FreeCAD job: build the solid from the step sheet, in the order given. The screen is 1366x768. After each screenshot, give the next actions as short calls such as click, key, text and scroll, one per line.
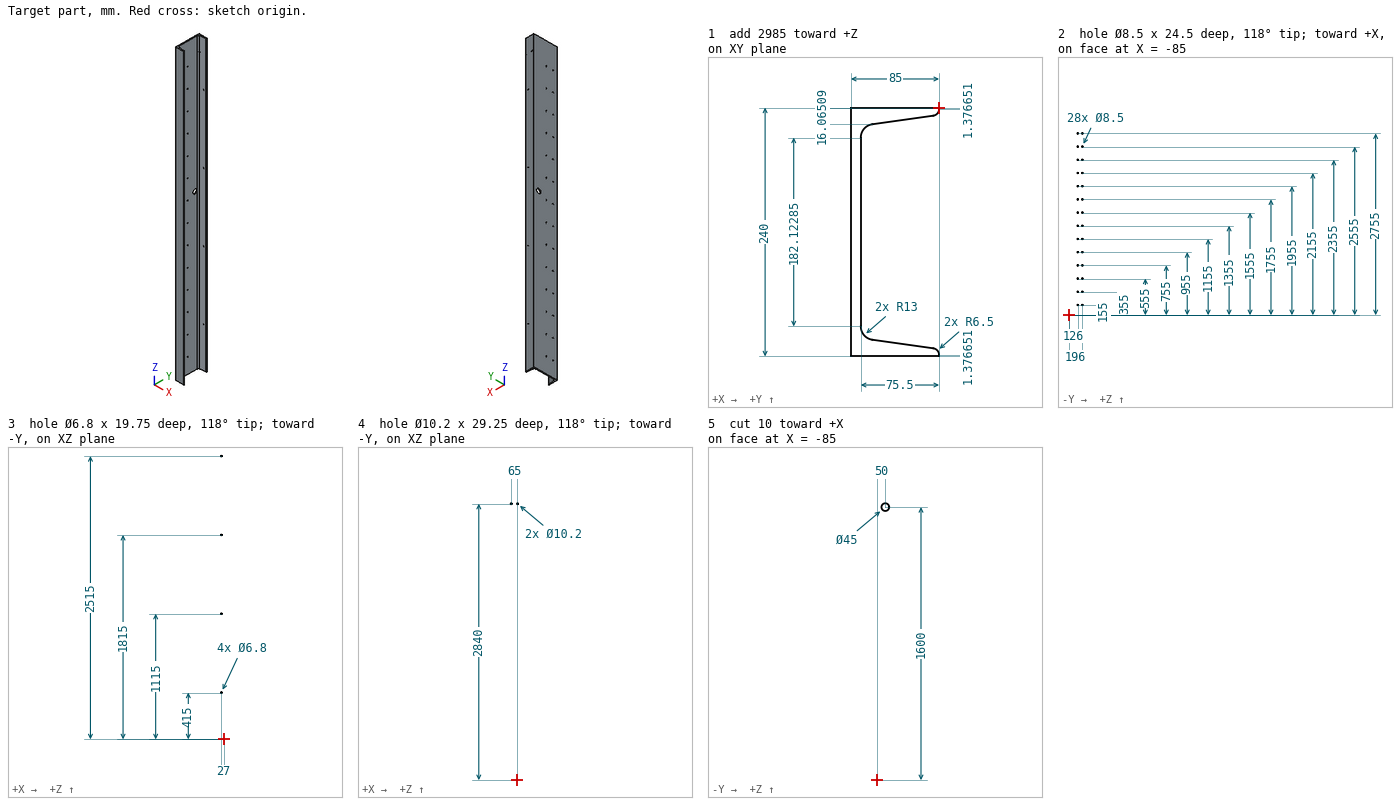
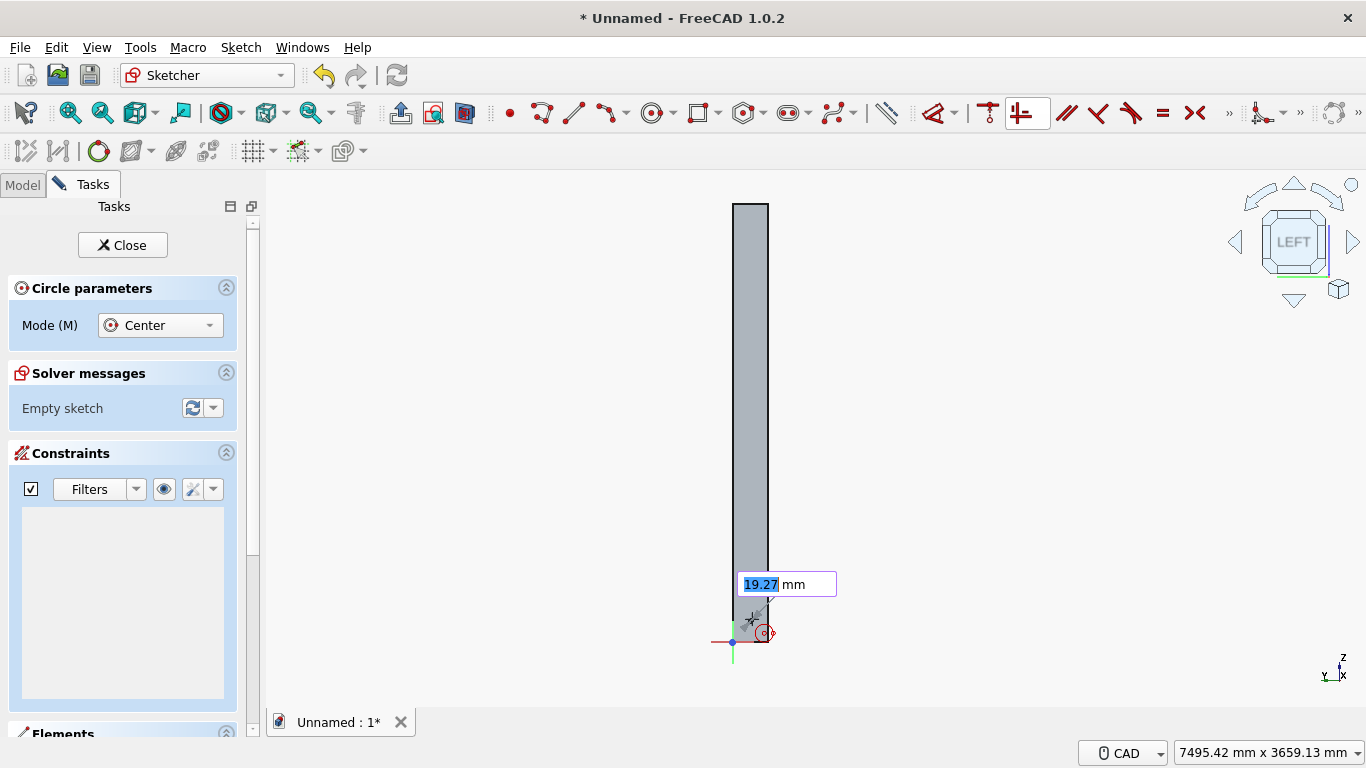
text(8.5)
key(Return)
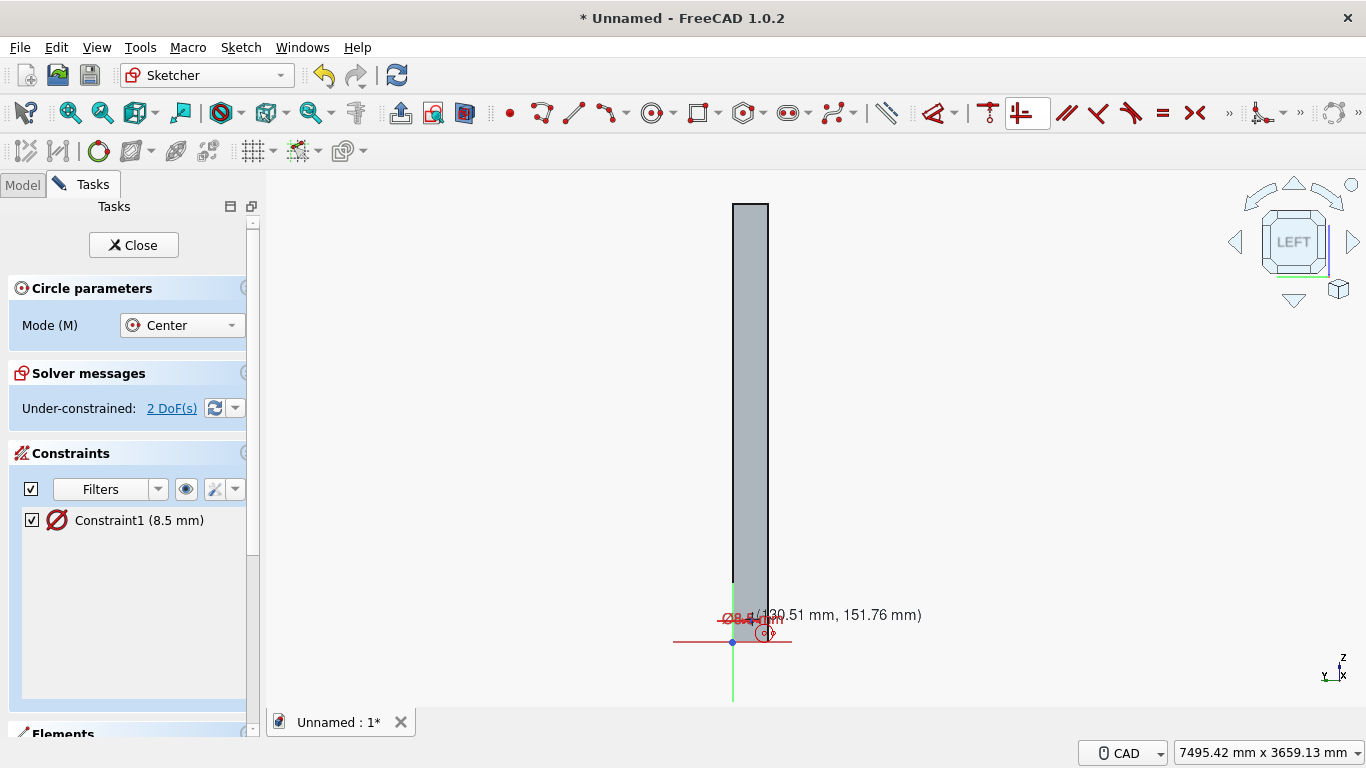
scroll(762, 620, up, 18)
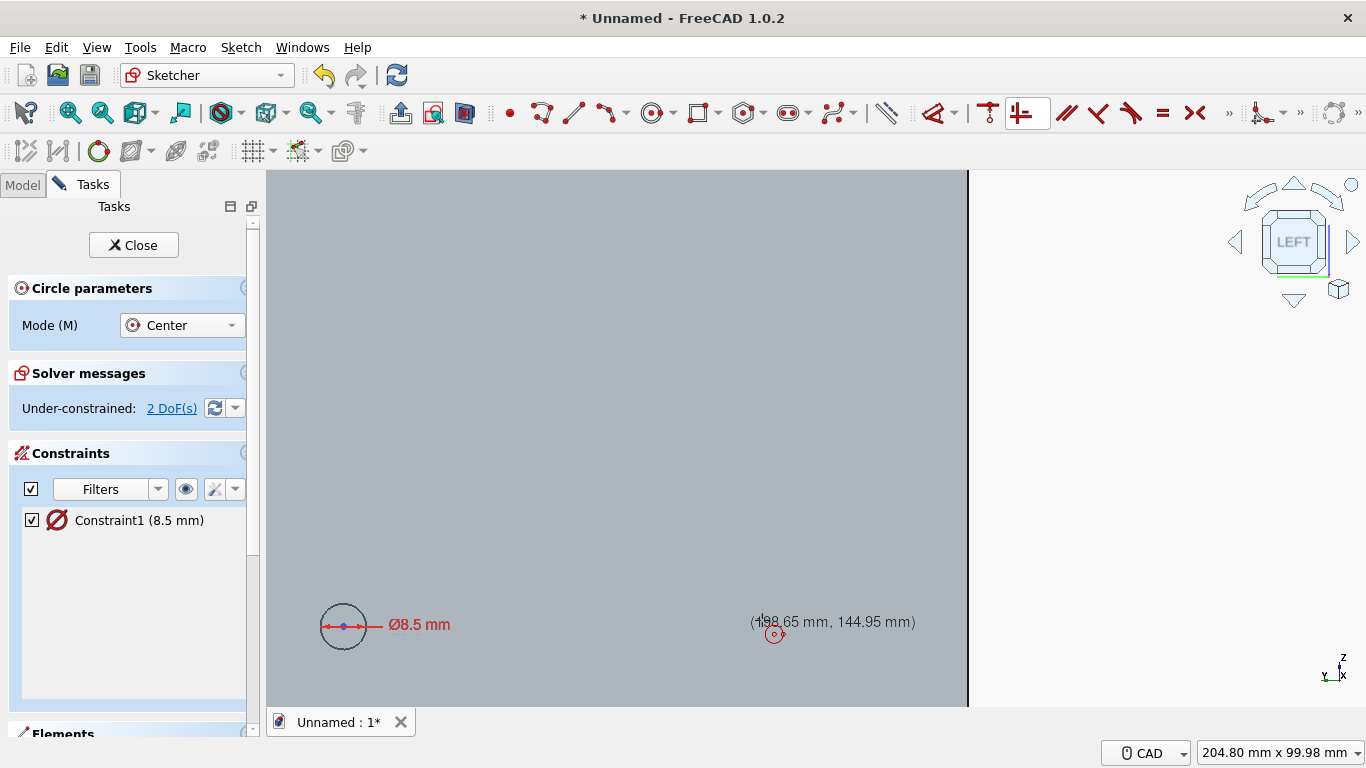
scroll(762, 619, down, 18)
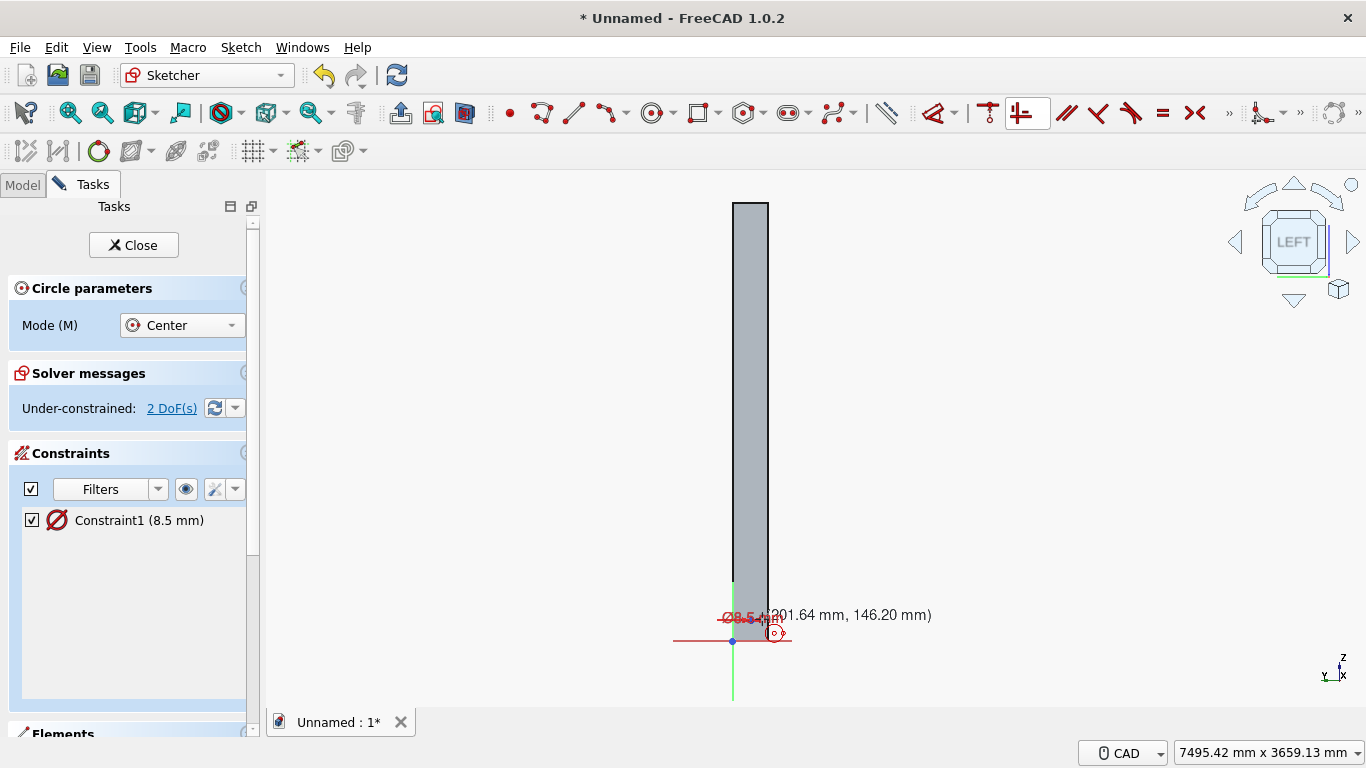
scroll(762, 619, up, 3)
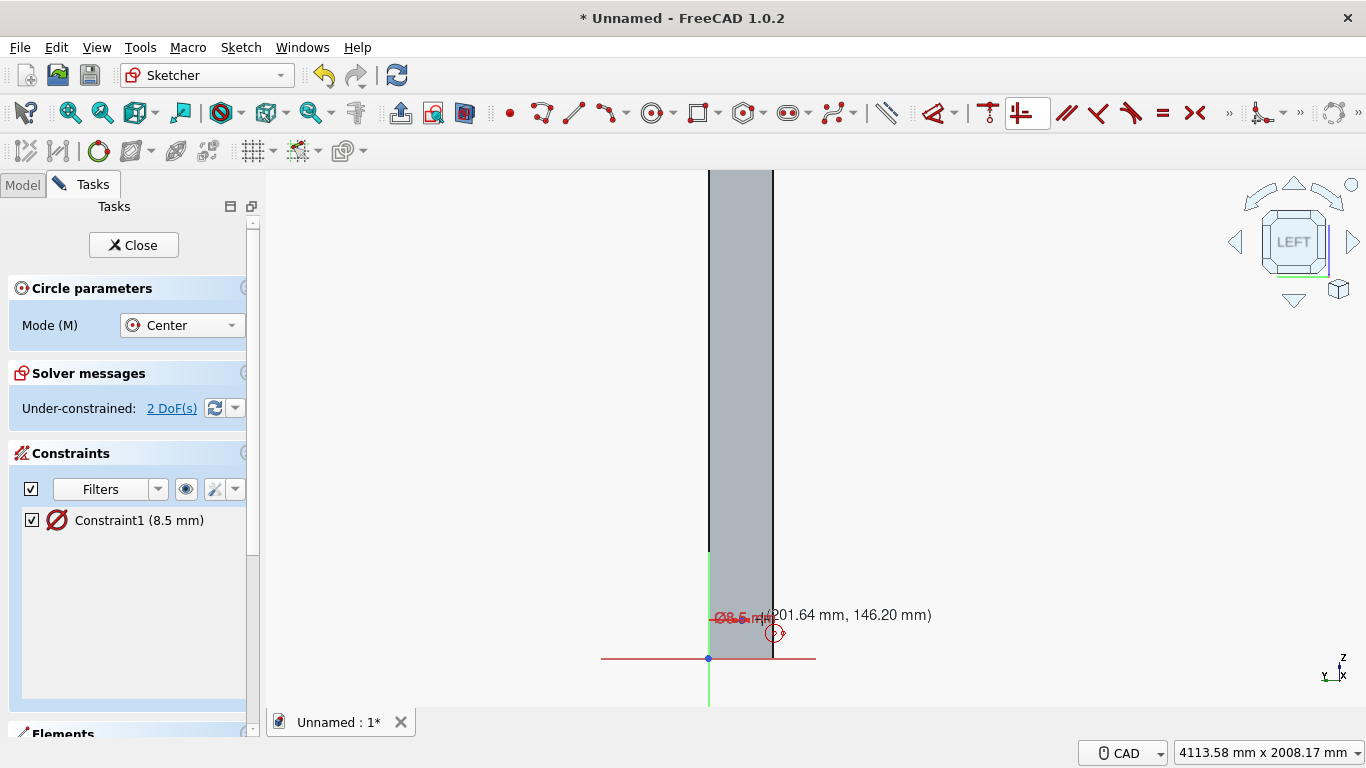
click(761, 617)
move(762, 617)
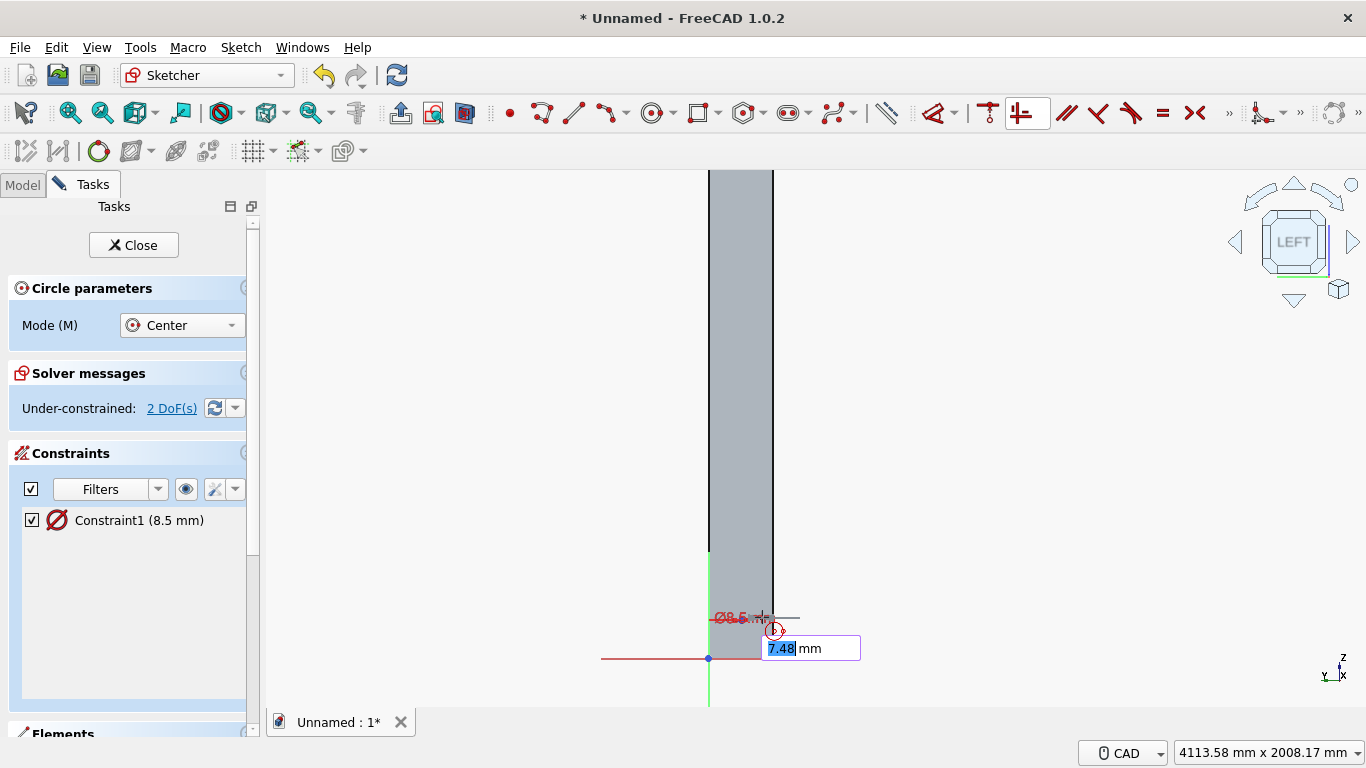
text(8.5)
key(Return)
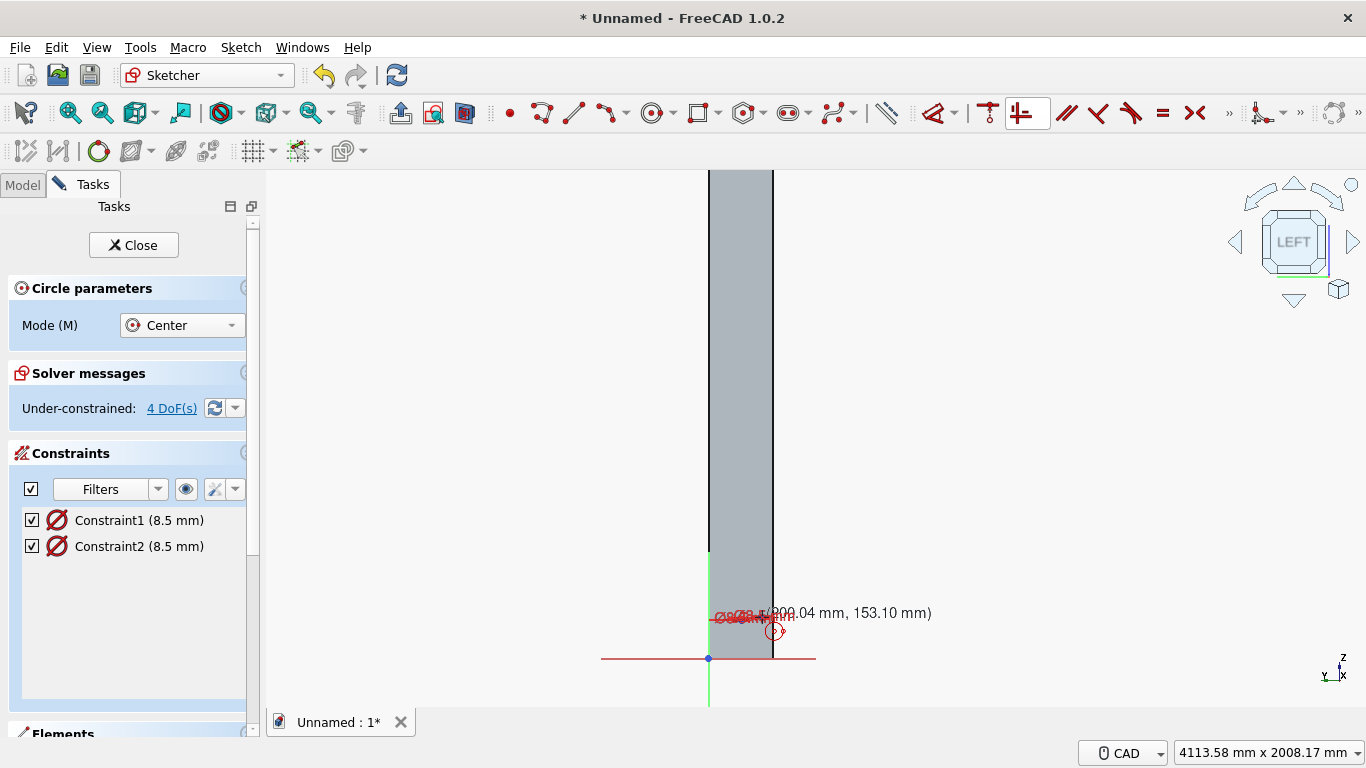
scroll(742, 564, up, 15)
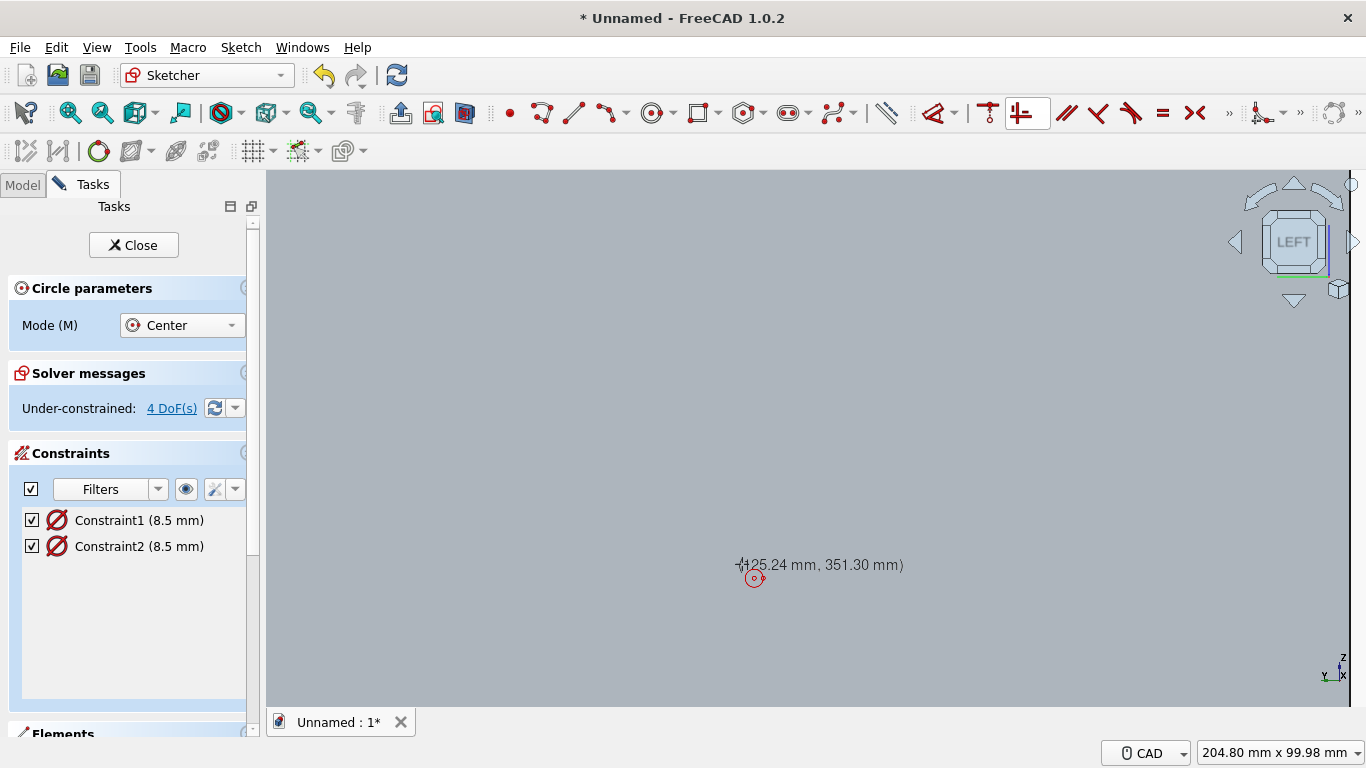
scroll(752, 590, down, 18)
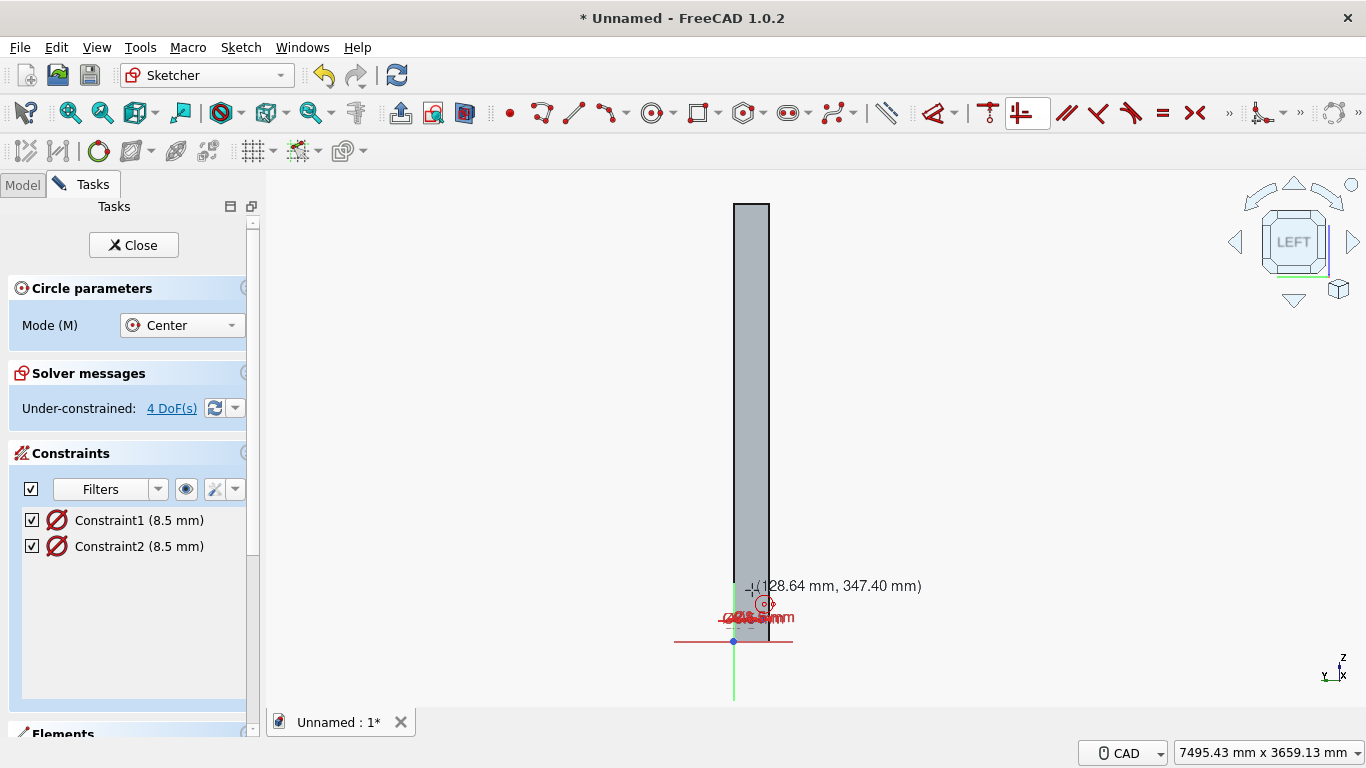
click(752, 590)
move(752, 589)